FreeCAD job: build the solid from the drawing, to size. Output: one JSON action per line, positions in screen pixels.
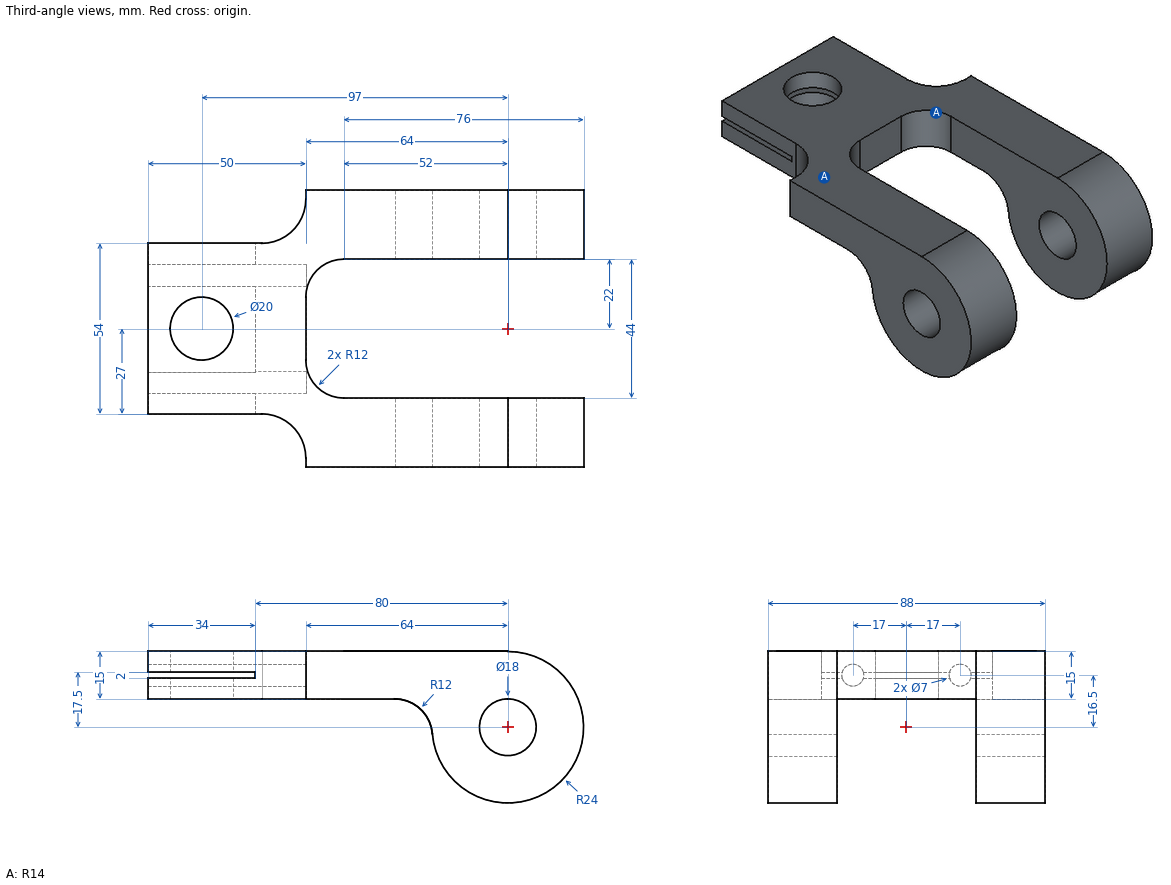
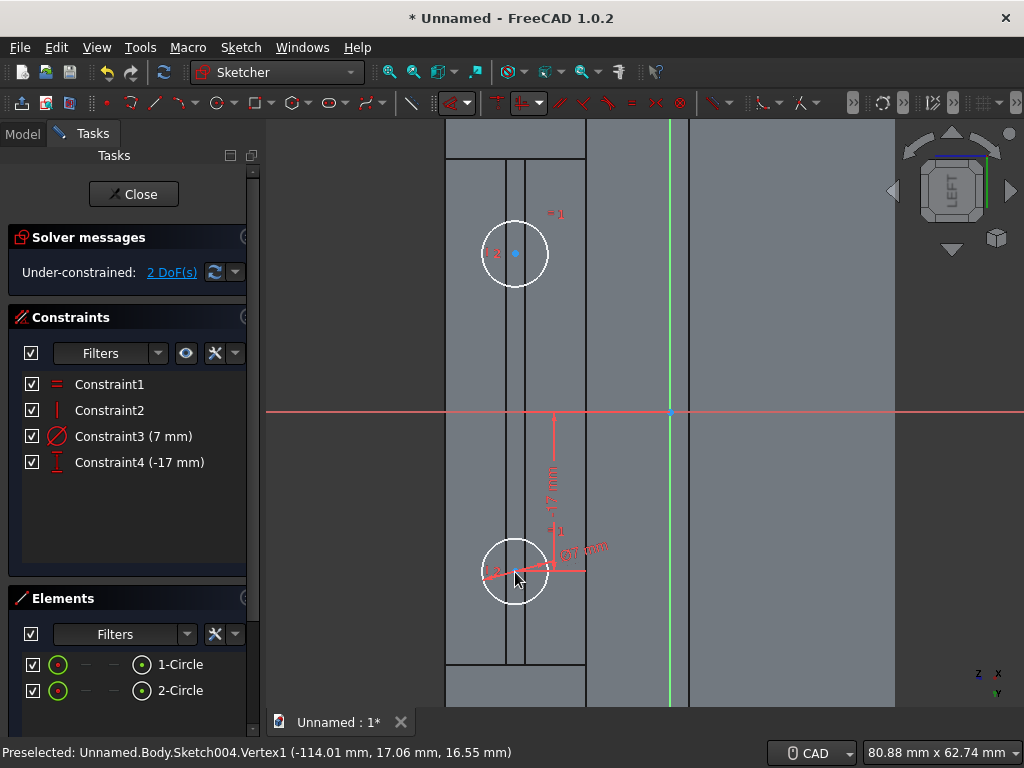
{"action": "left_click", "coordinate": [515, 254]}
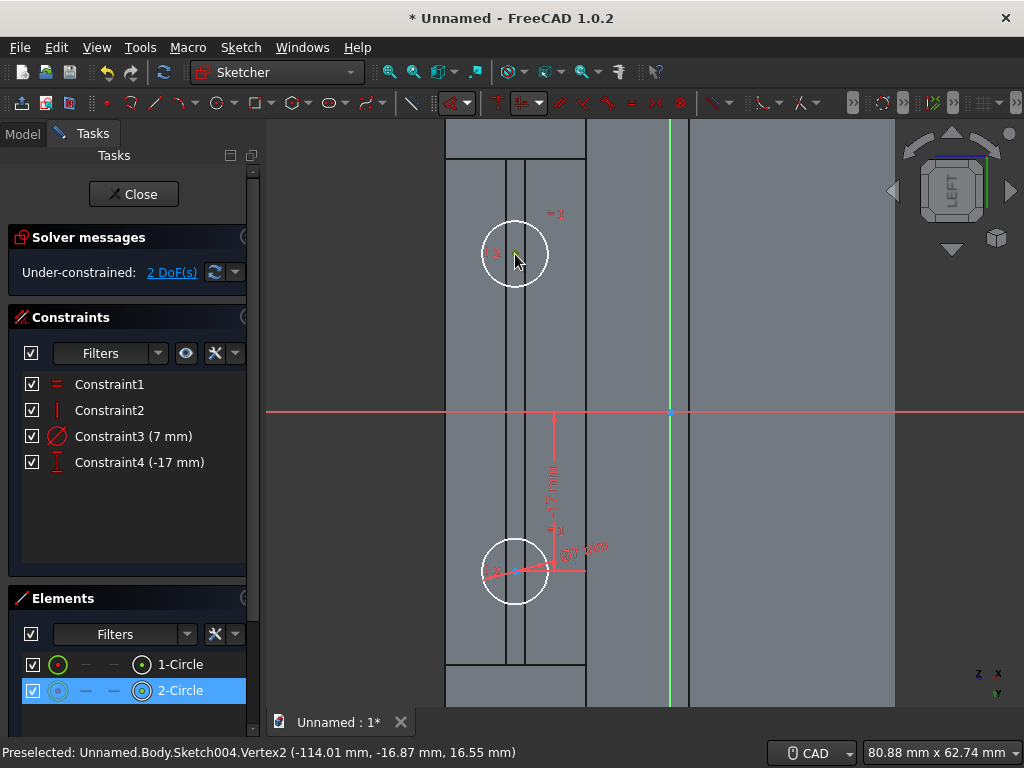
{"action": "left_click", "coordinate": [470, 104]}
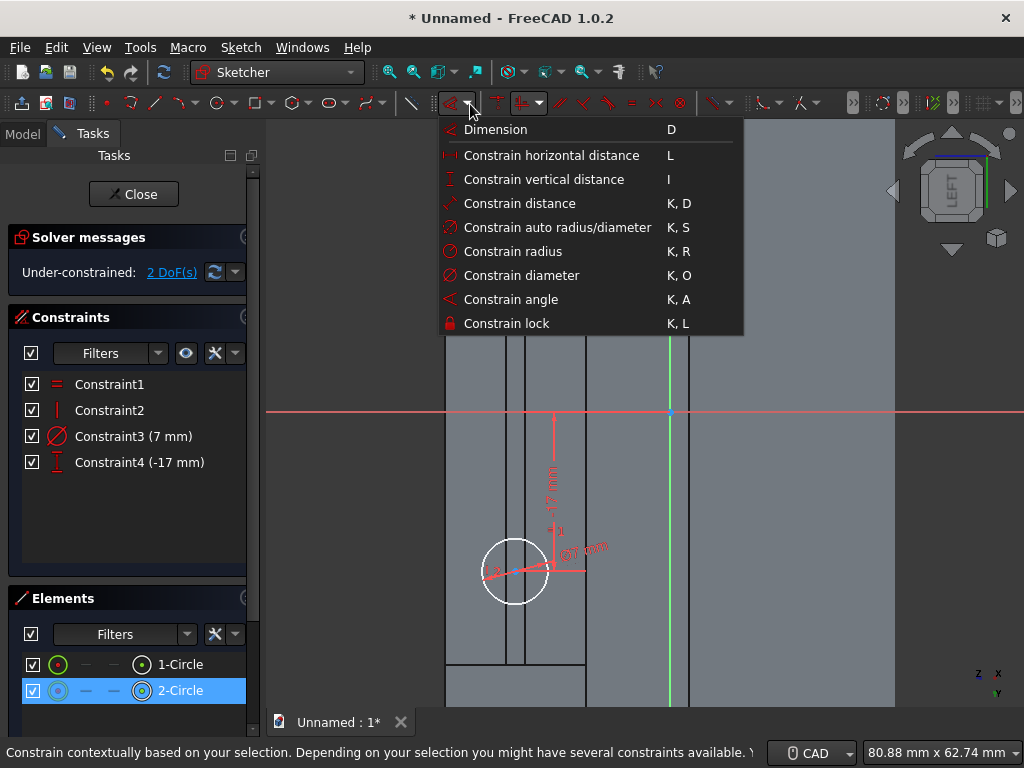
{"action": "left_click", "coordinate": [591, 179]}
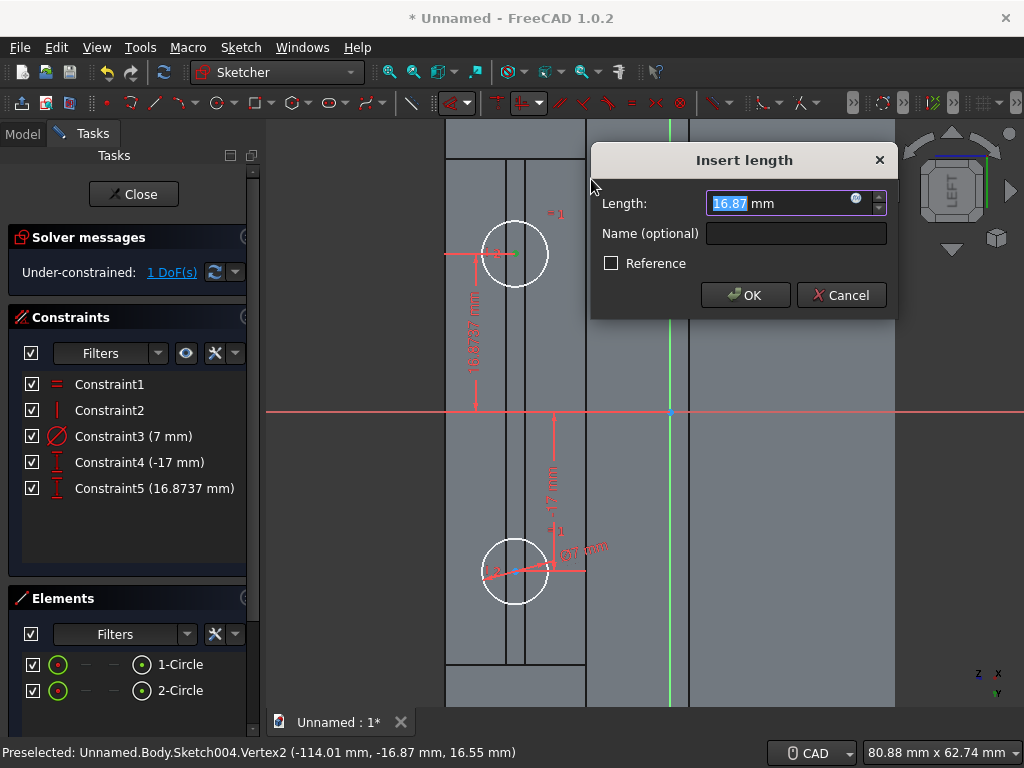
{"action": "type", "text": "17"}
{"action": "key", "text": "Return"}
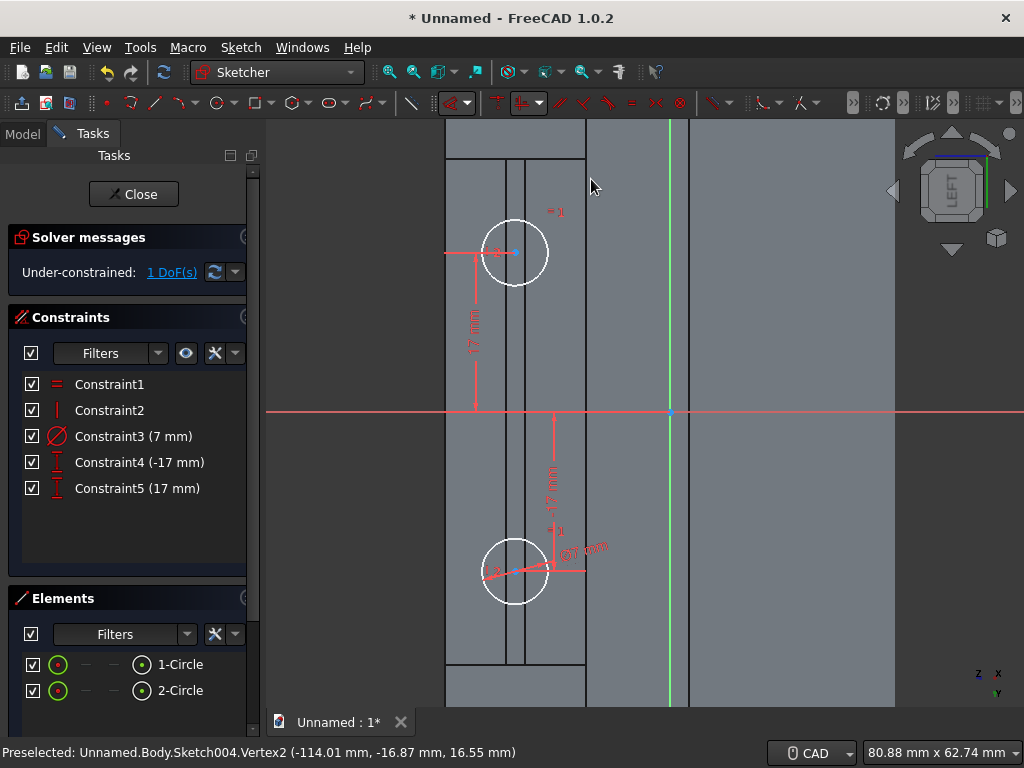
{"action": "left_click", "coordinate": [515, 571]}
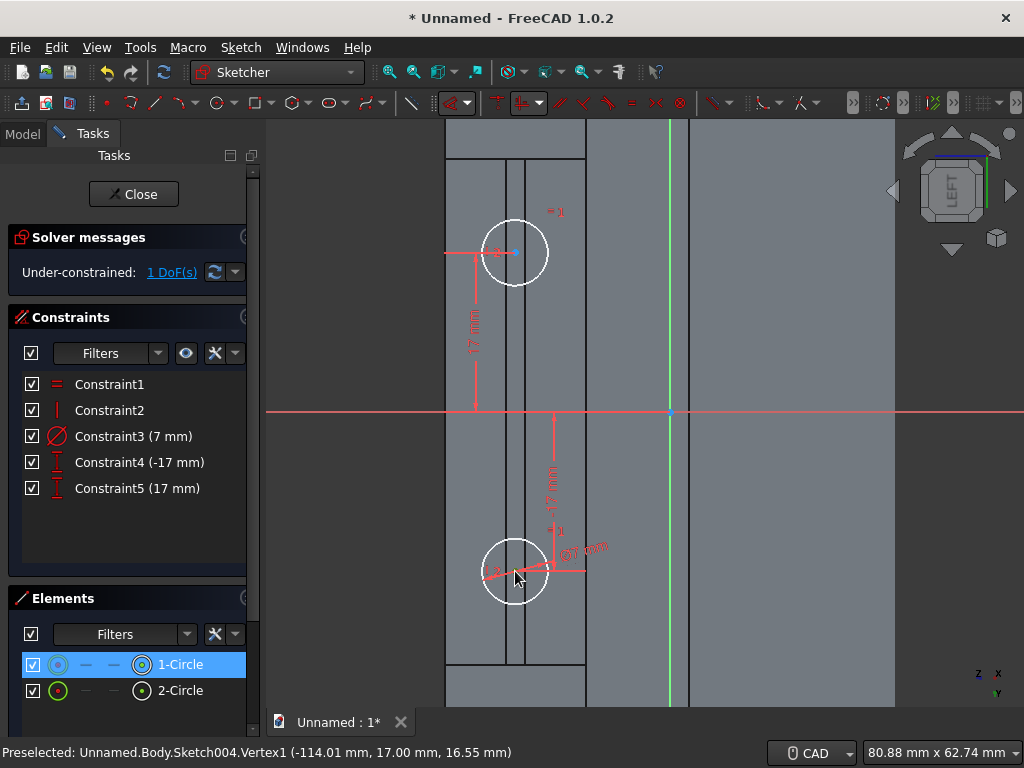
{"action": "left_click", "coordinate": [470, 104]}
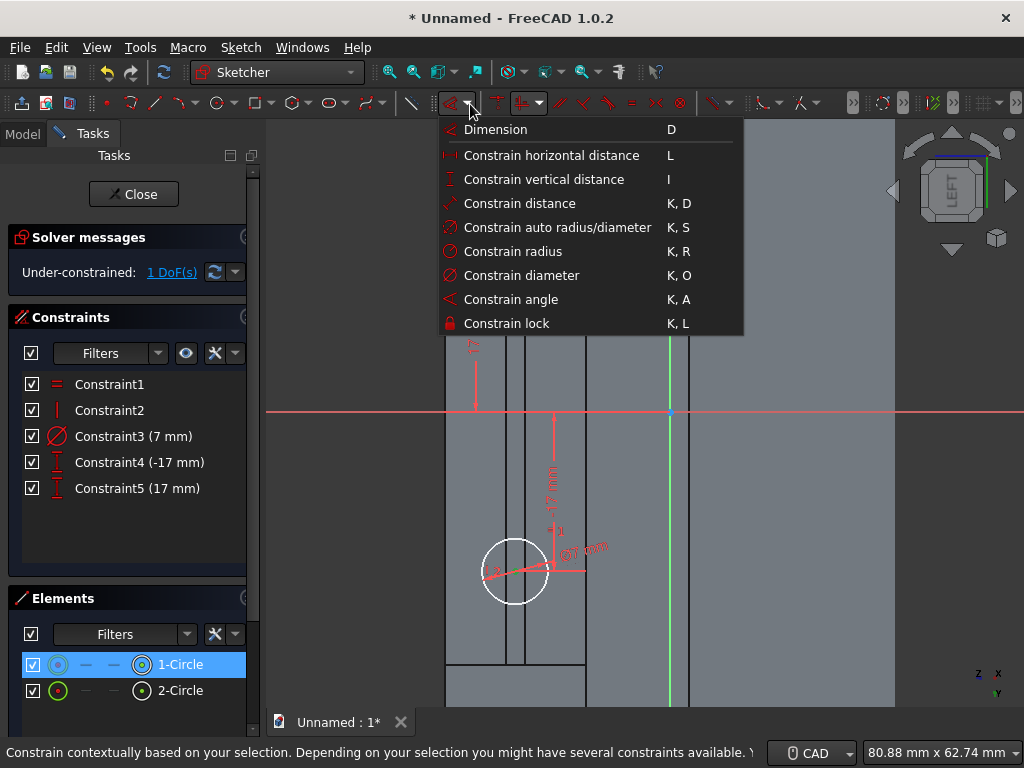
{"action": "left_click", "coordinate": [591, 155]}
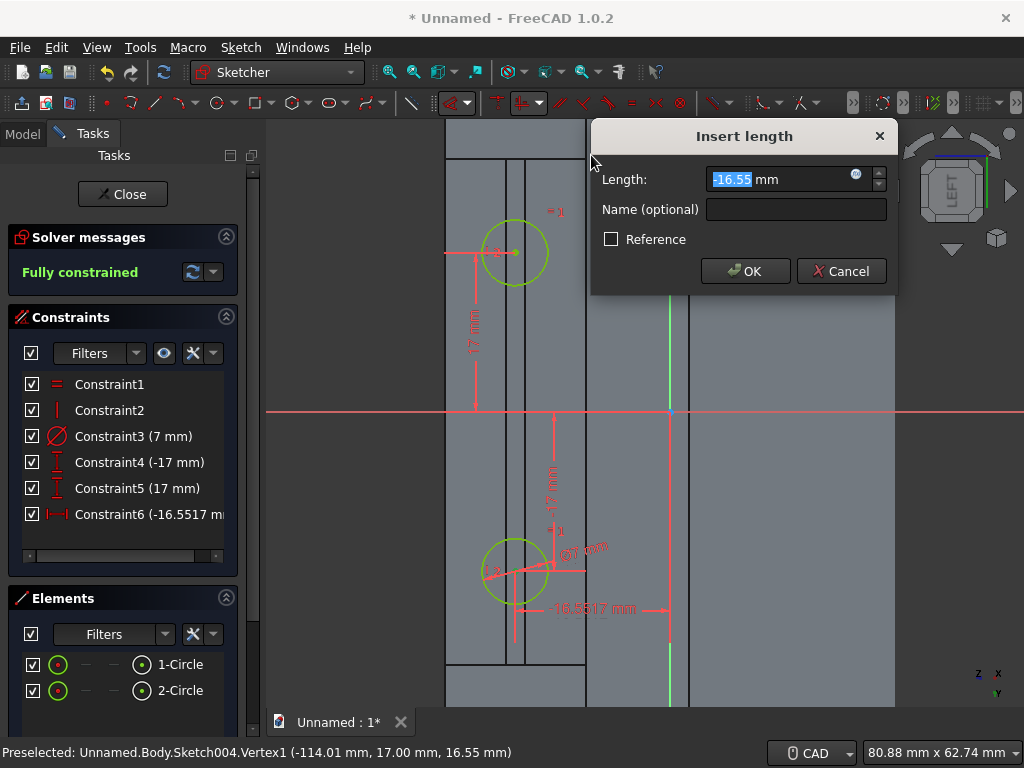
{"action": "type", "text": "-16.5"}
{"action": "key", "text": "Return"}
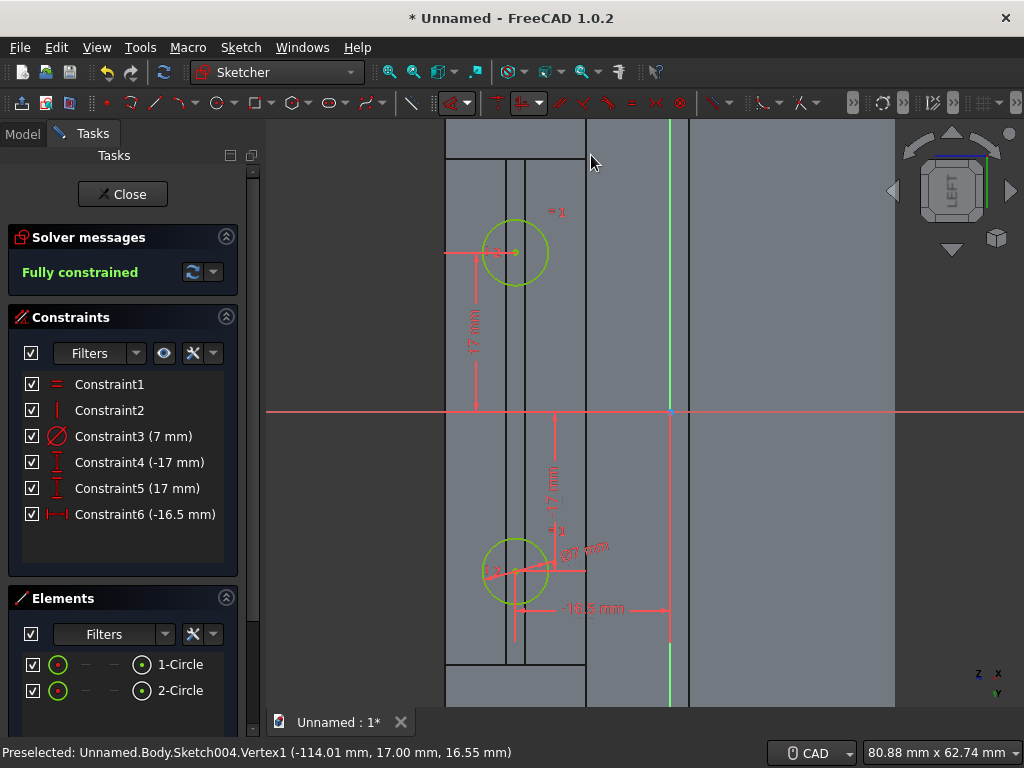
{"action": "left_click", "coordinate": [123, 194]}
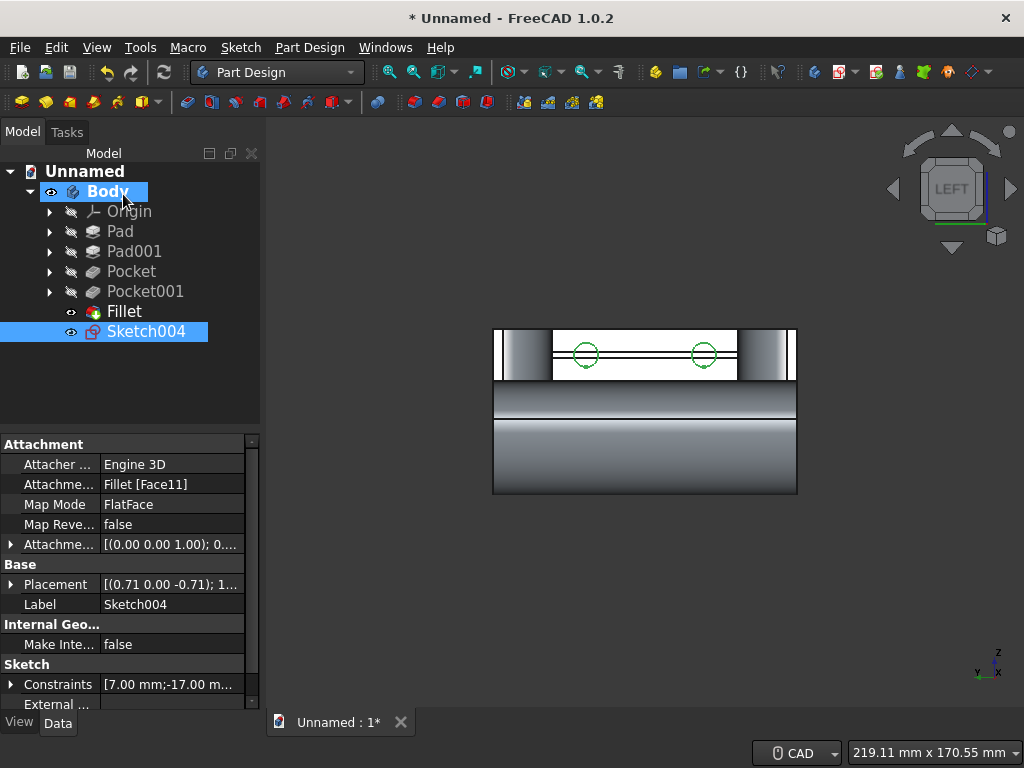
{"action": "left_click", "coordinate": [188, 102]}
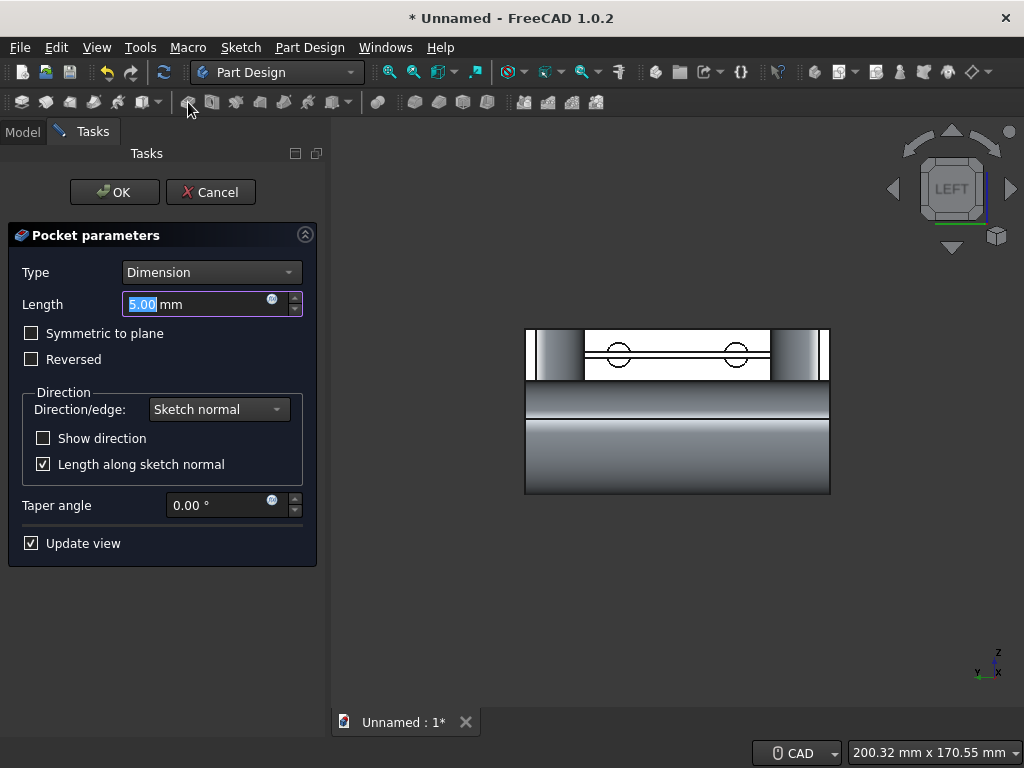
{"action": "type", "text": "50"}
{"action": "key", "text": "Tab"}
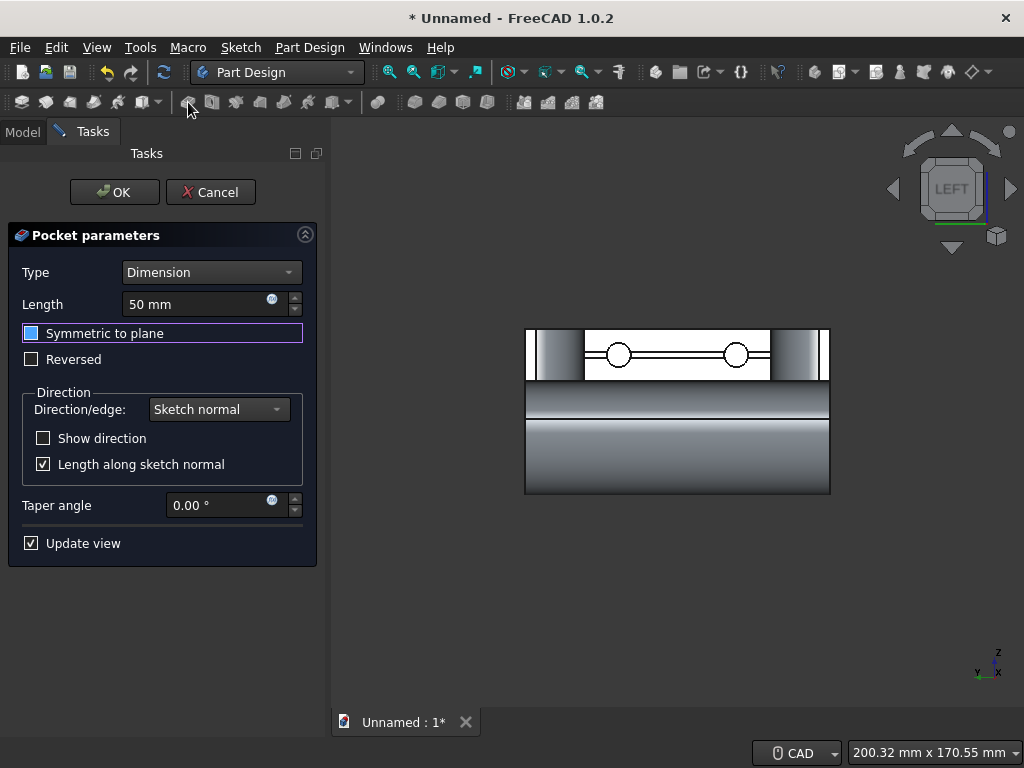
{"action": "left_click", "coordinate": [115, 192]}